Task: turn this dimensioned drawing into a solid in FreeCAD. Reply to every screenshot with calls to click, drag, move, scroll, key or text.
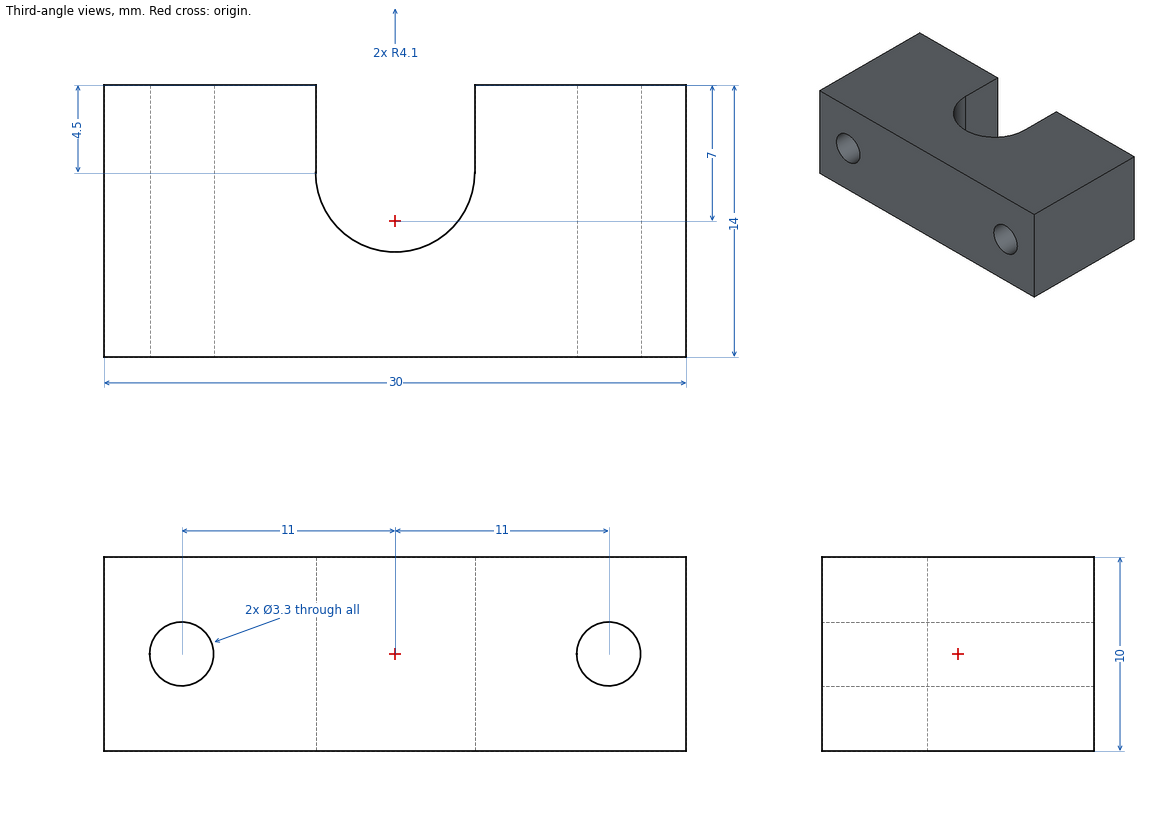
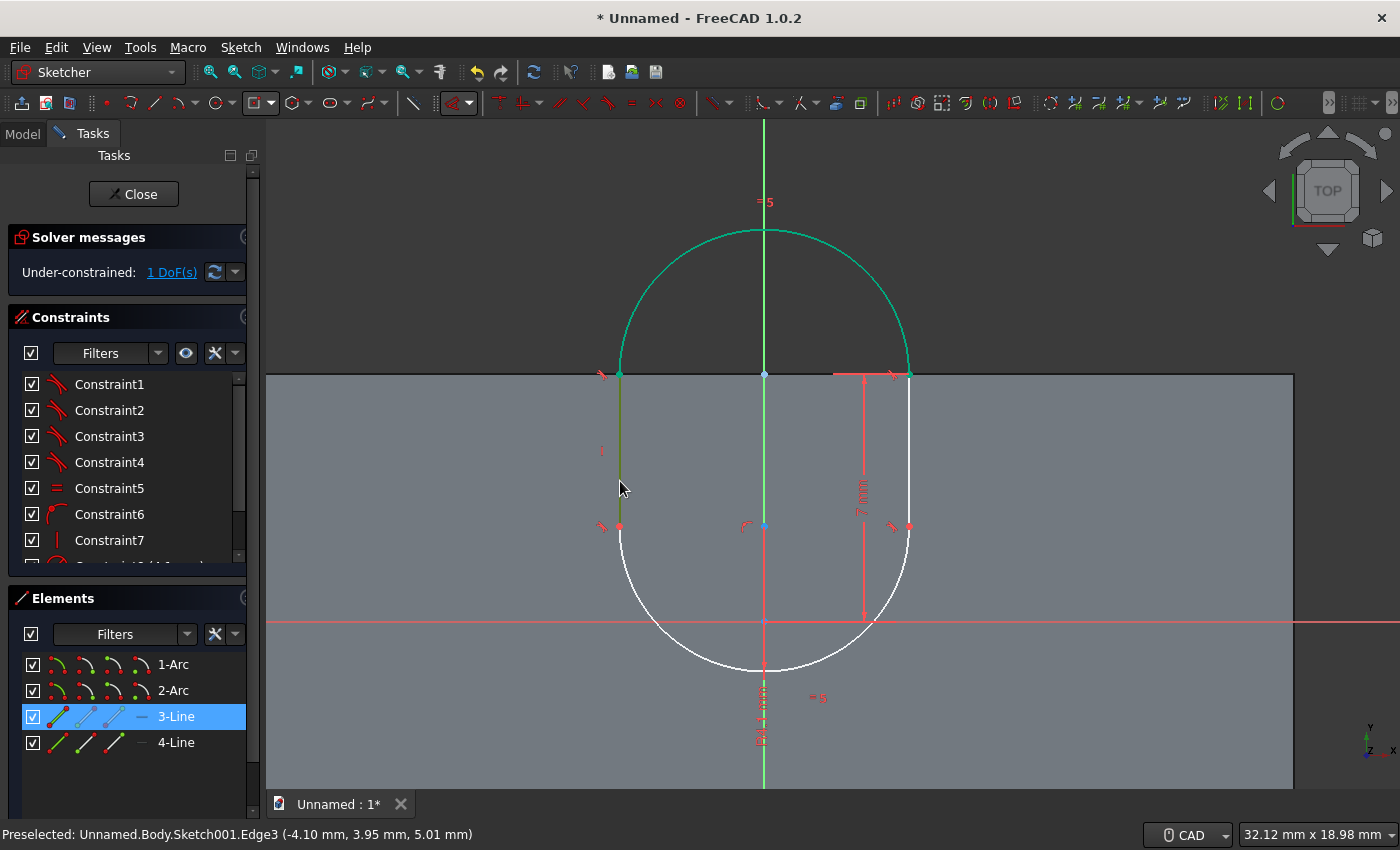
click(472, 104)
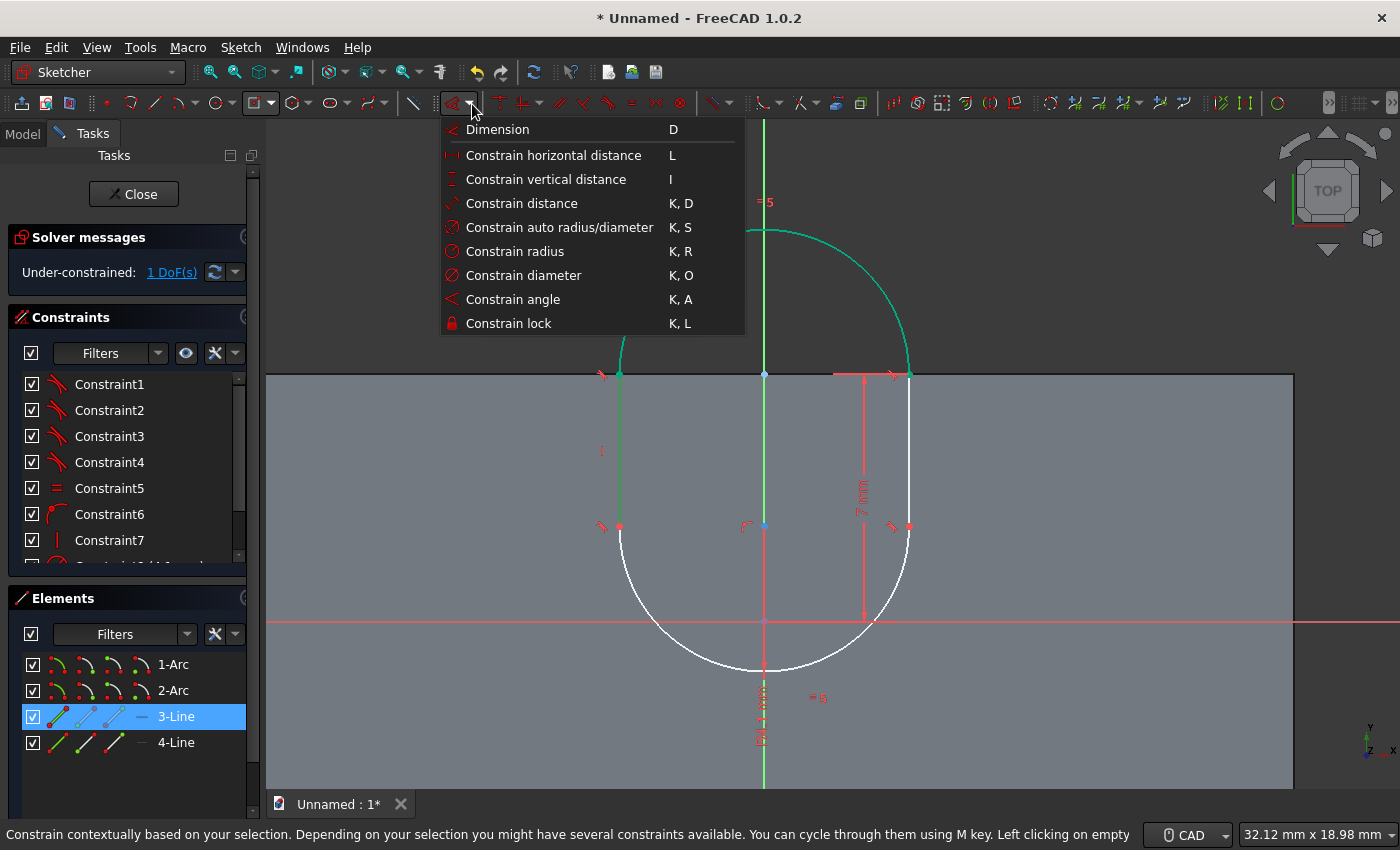
click(593, 179)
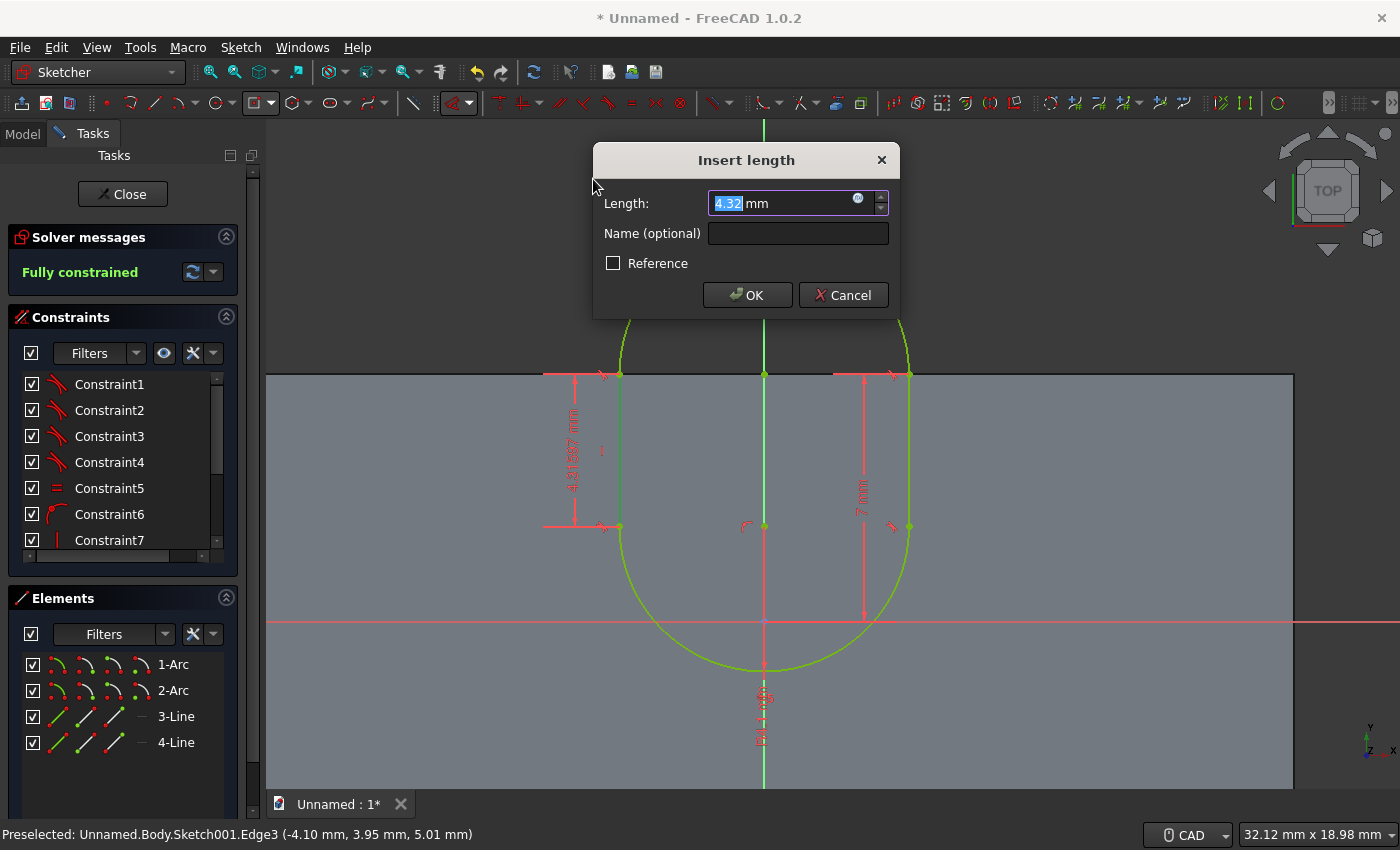
text(4.5)
key(Return)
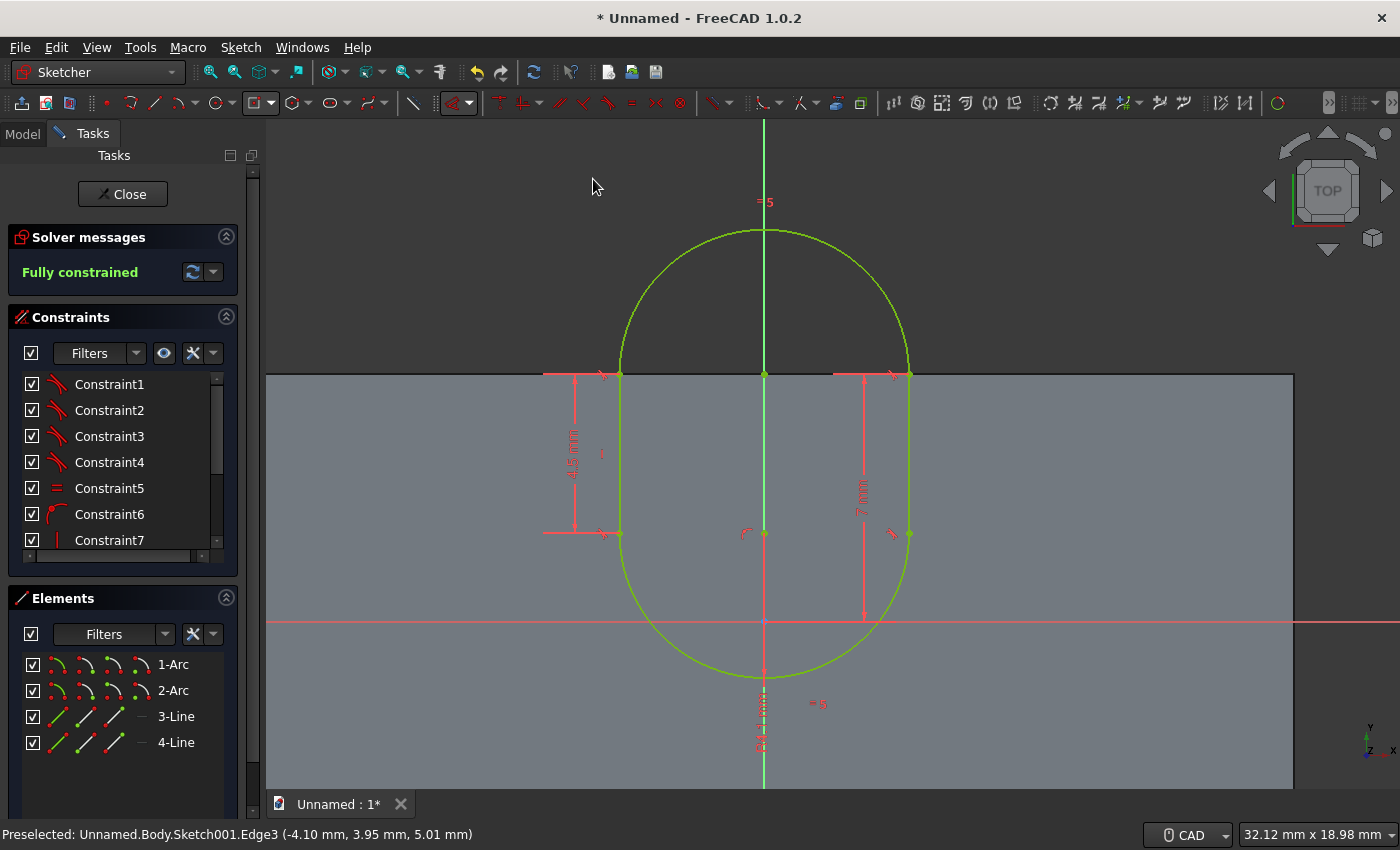
click(123, 194)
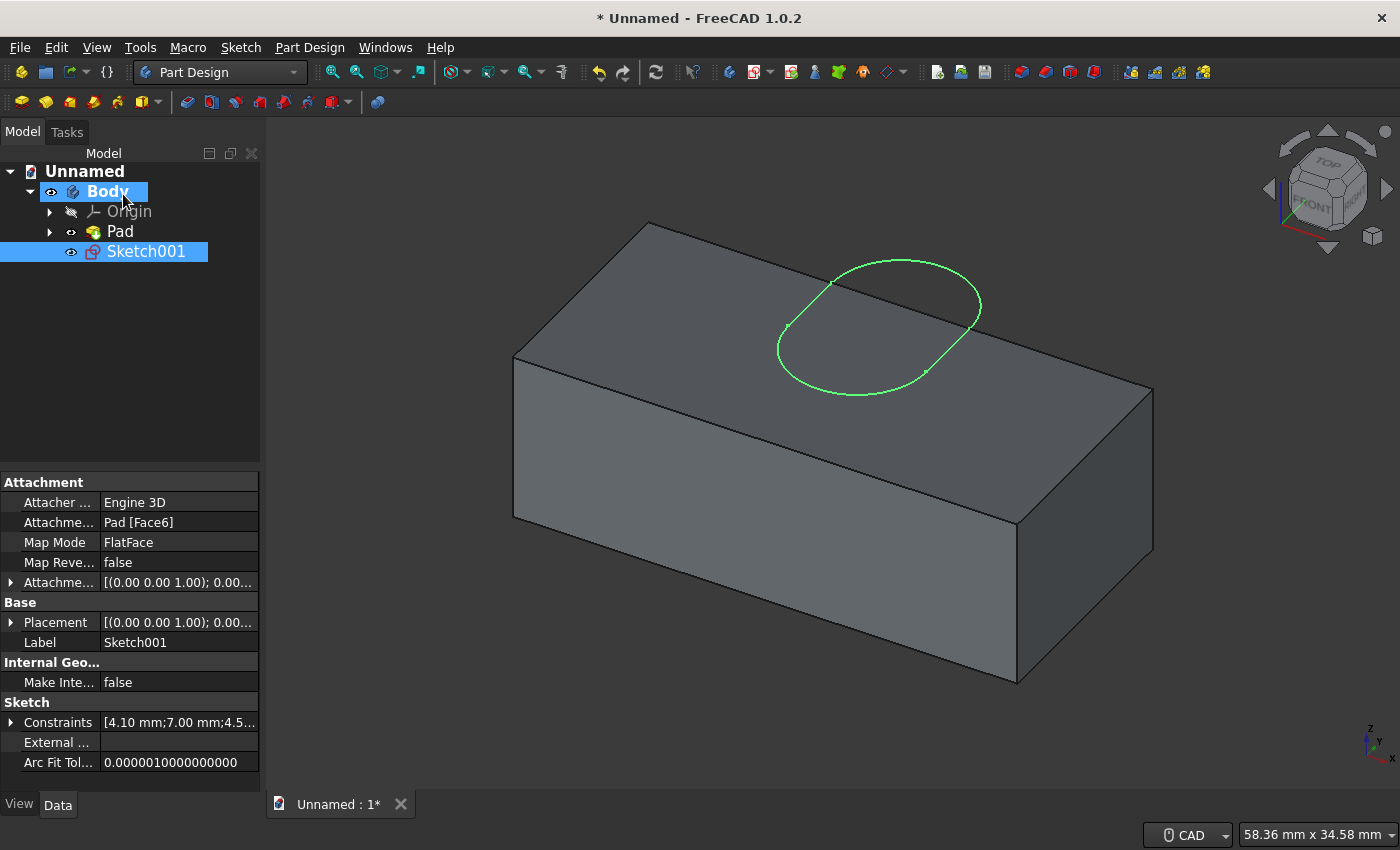
click(188, 102)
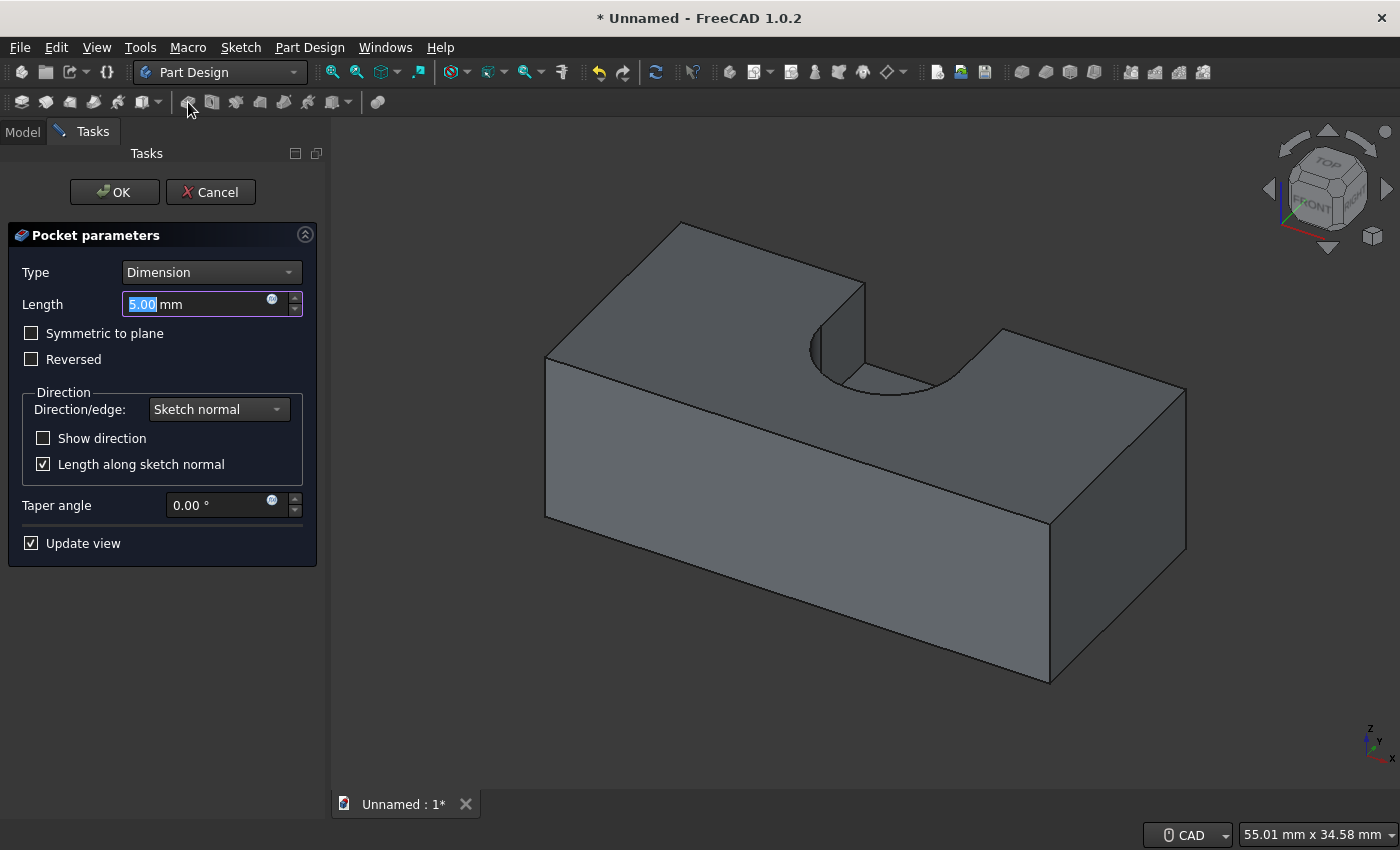
click(212, 272)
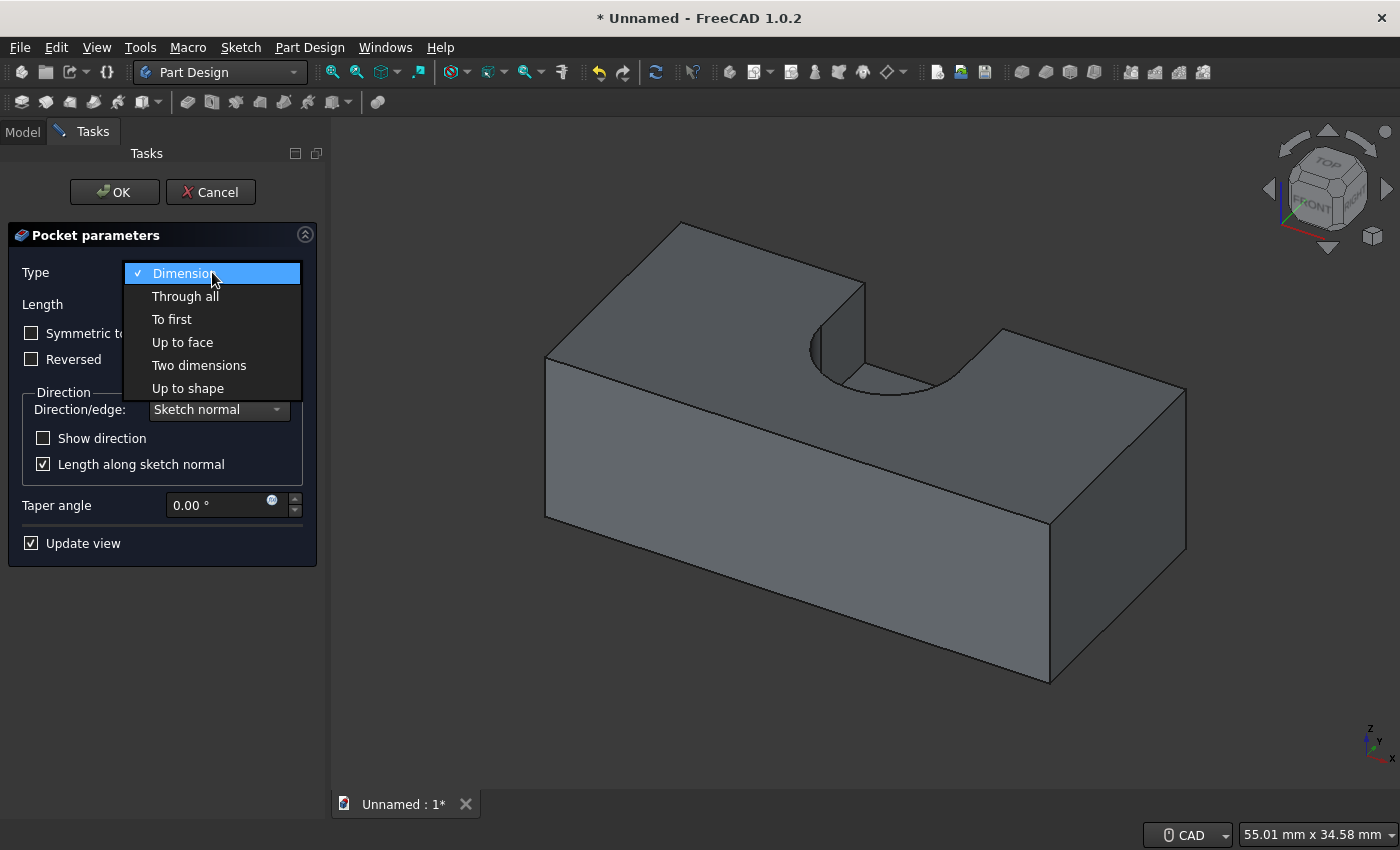
click(212, 296)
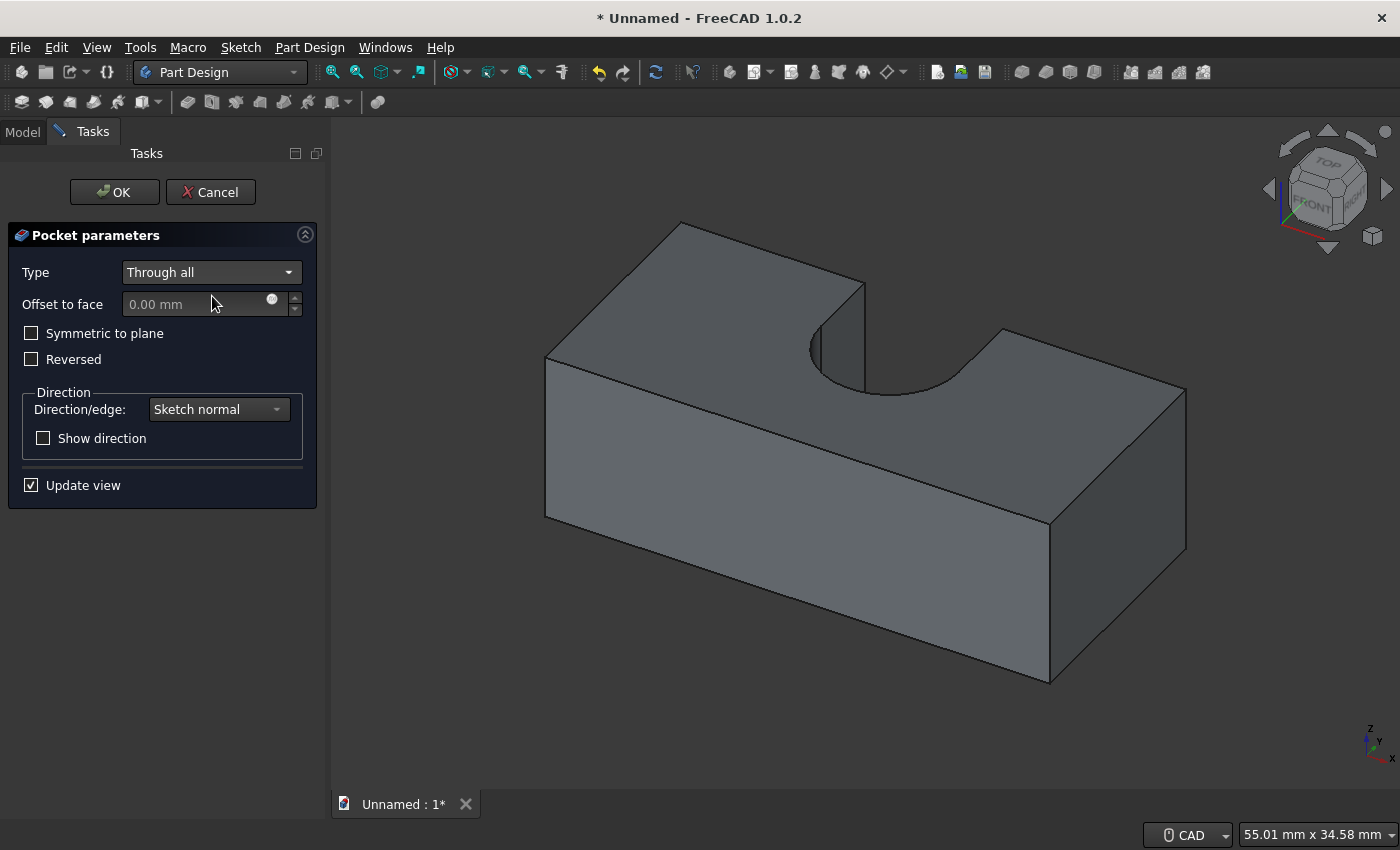
click(115, 192)